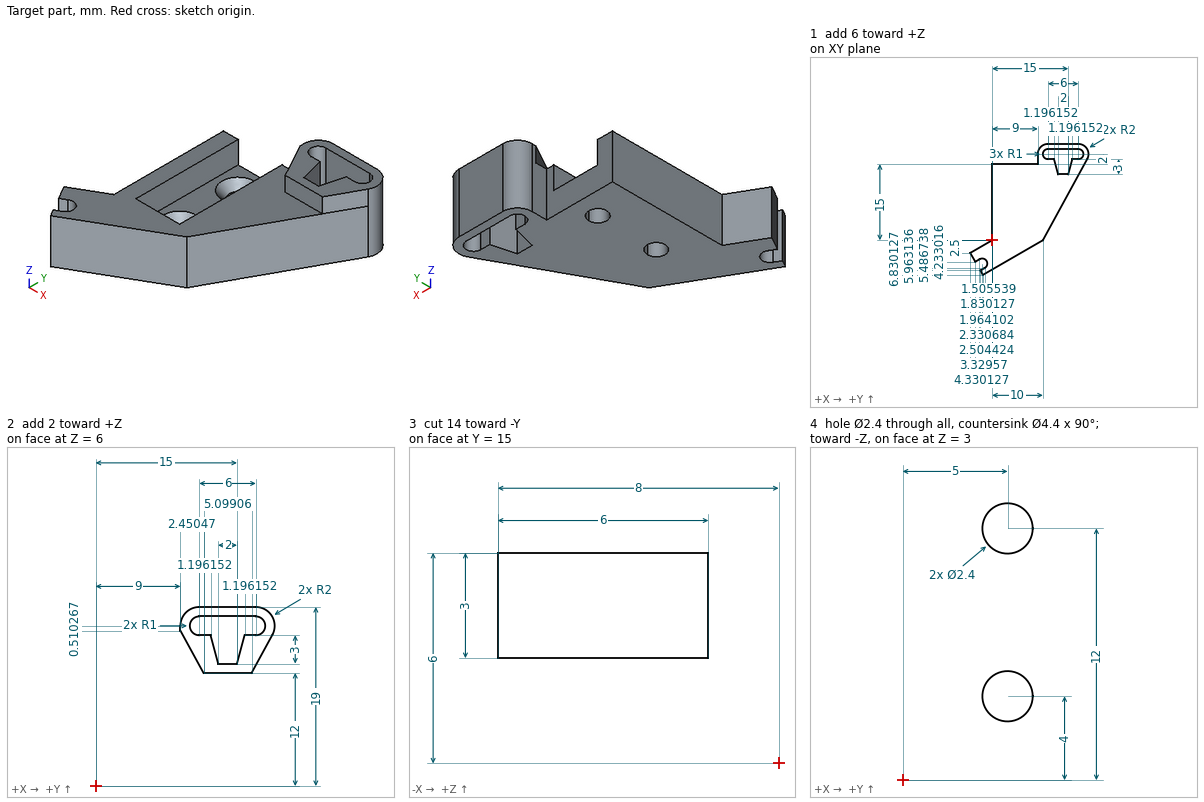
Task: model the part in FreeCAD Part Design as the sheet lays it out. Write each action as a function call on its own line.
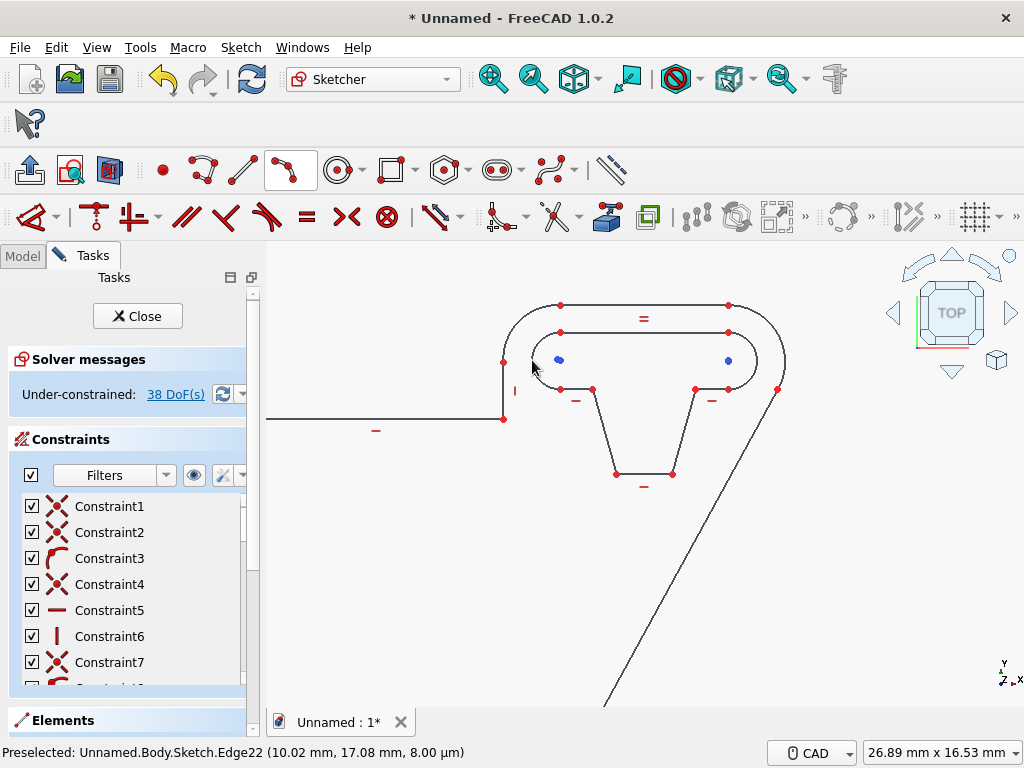
click(704, 524)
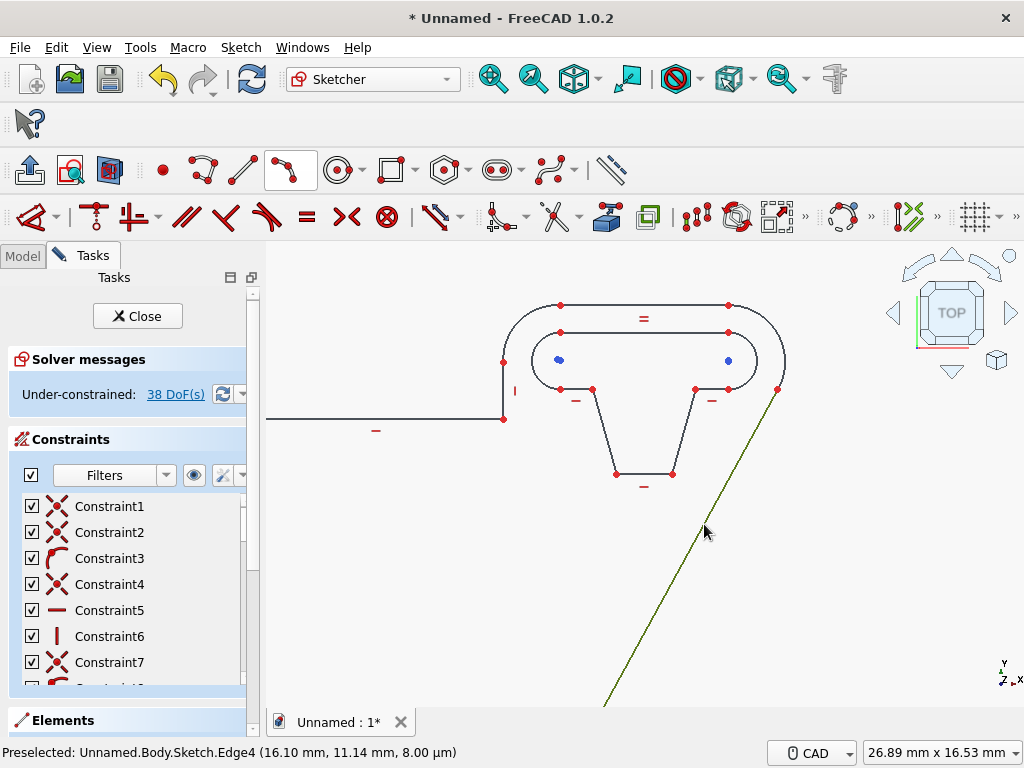
click(785, 356)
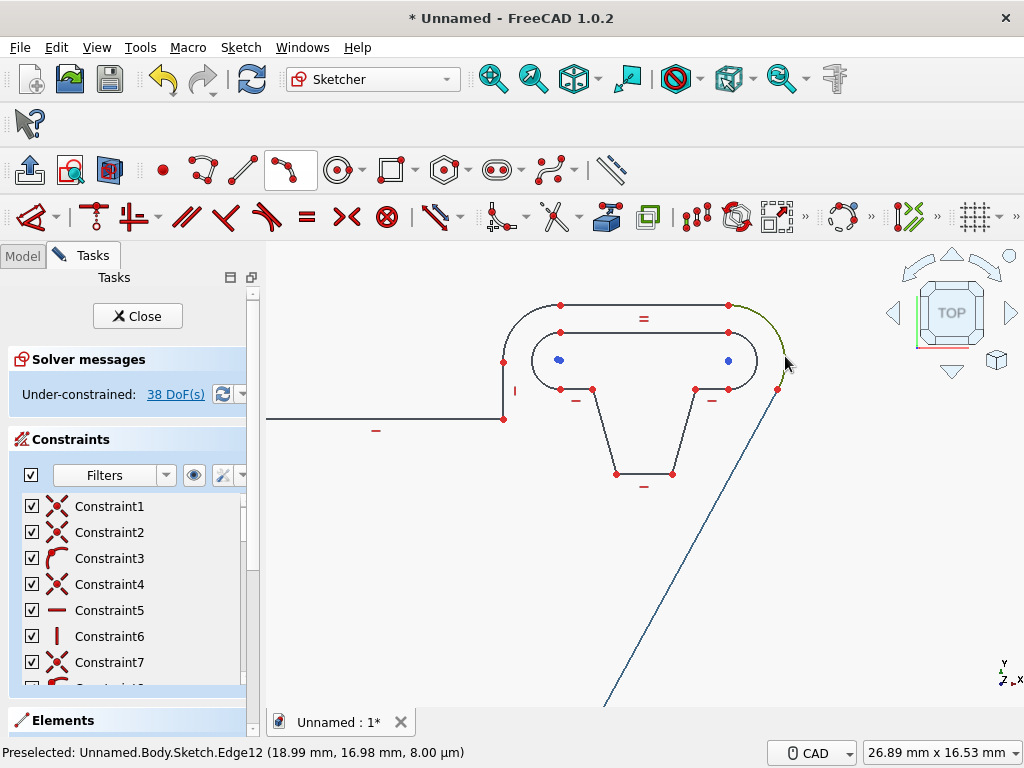
key(t)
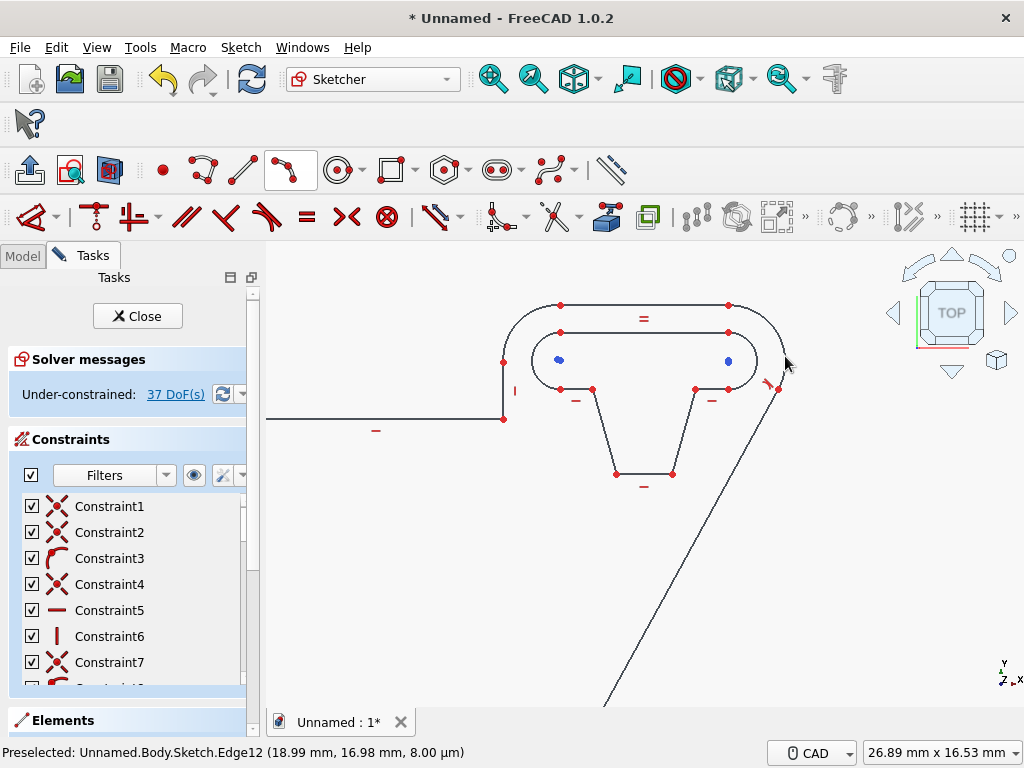
click(678, 305)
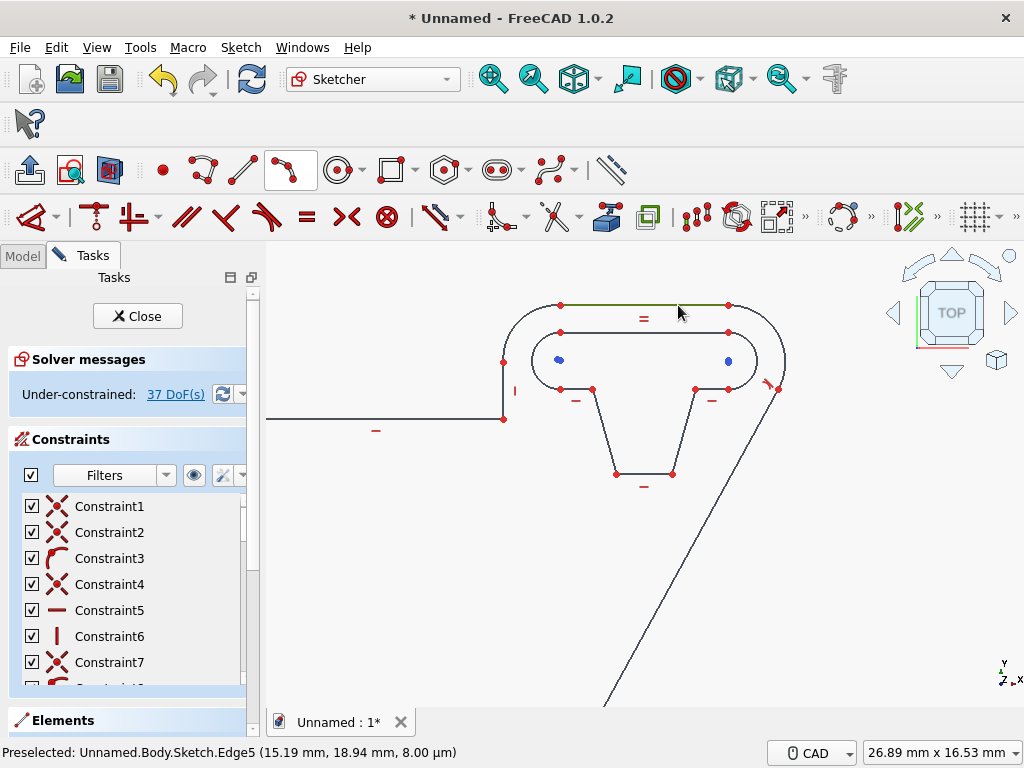
click(785, 355)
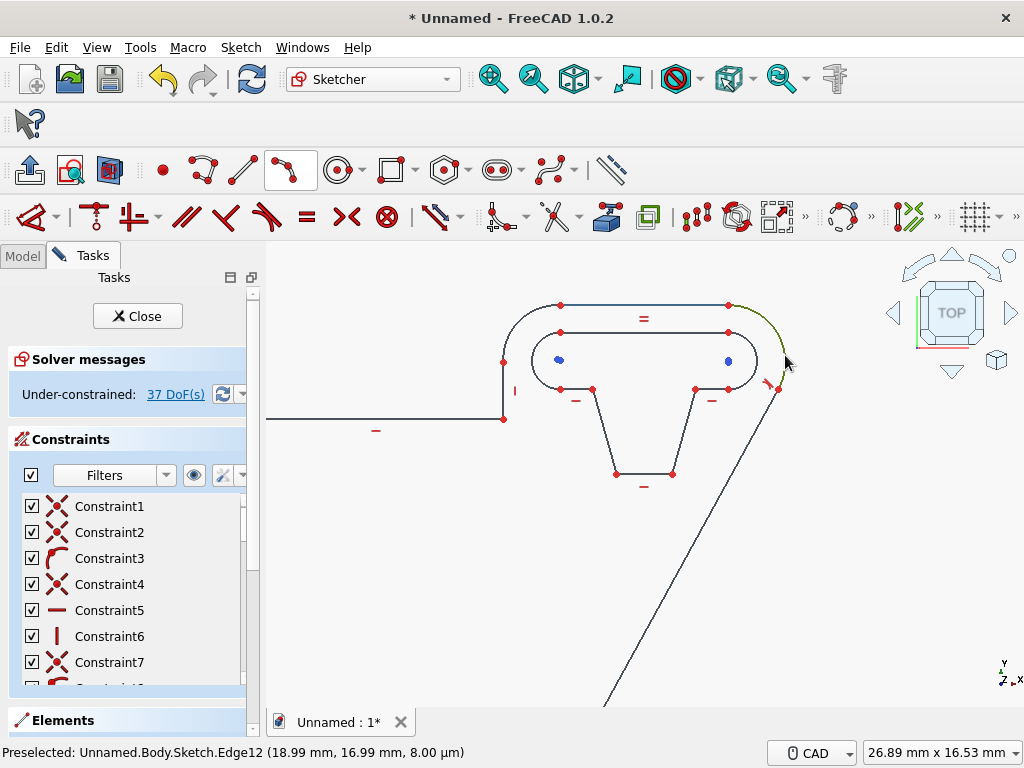
click(268, 218)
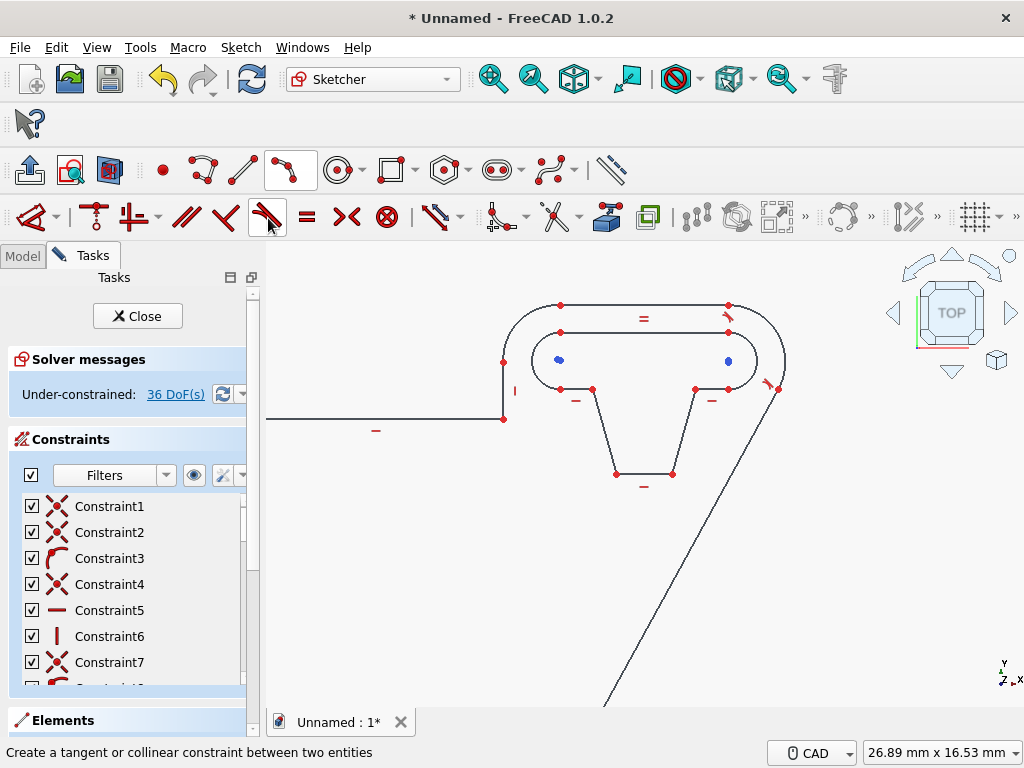
click(678, 305)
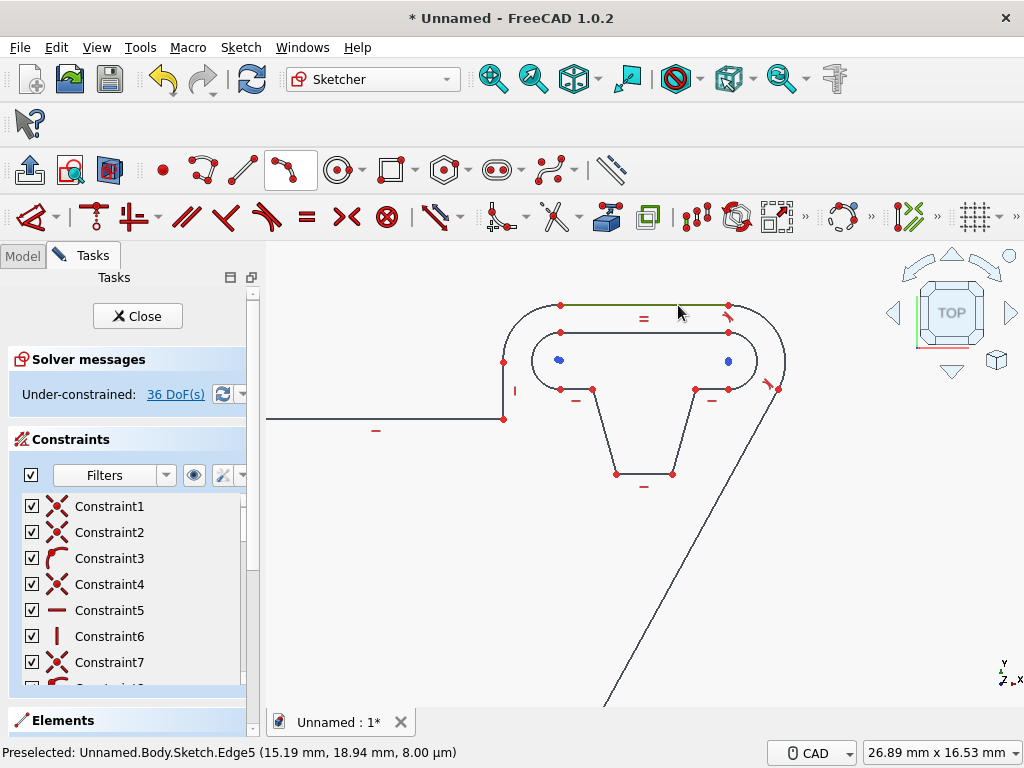
click(534, 311)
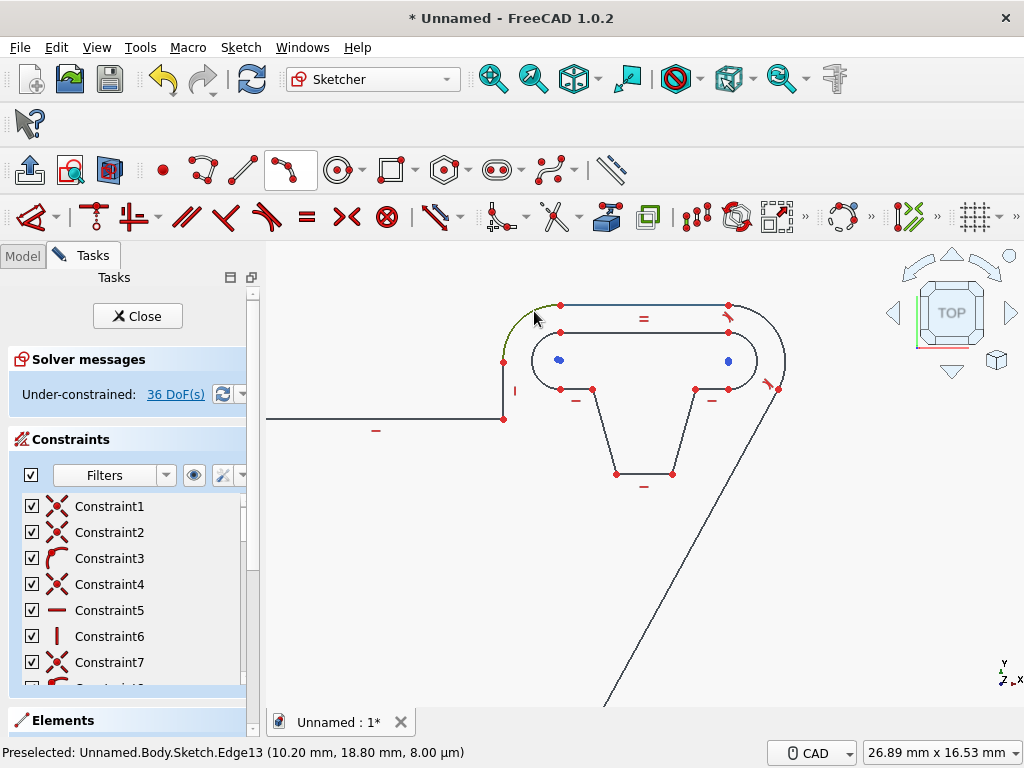
click(268, 218)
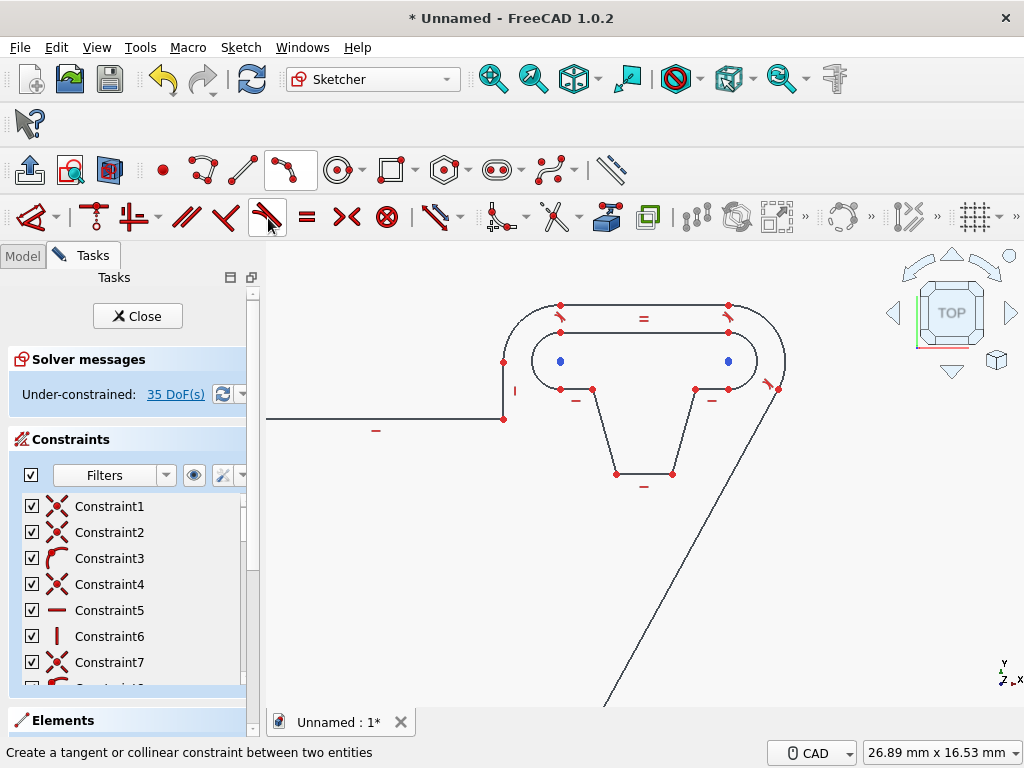
click(503, 379)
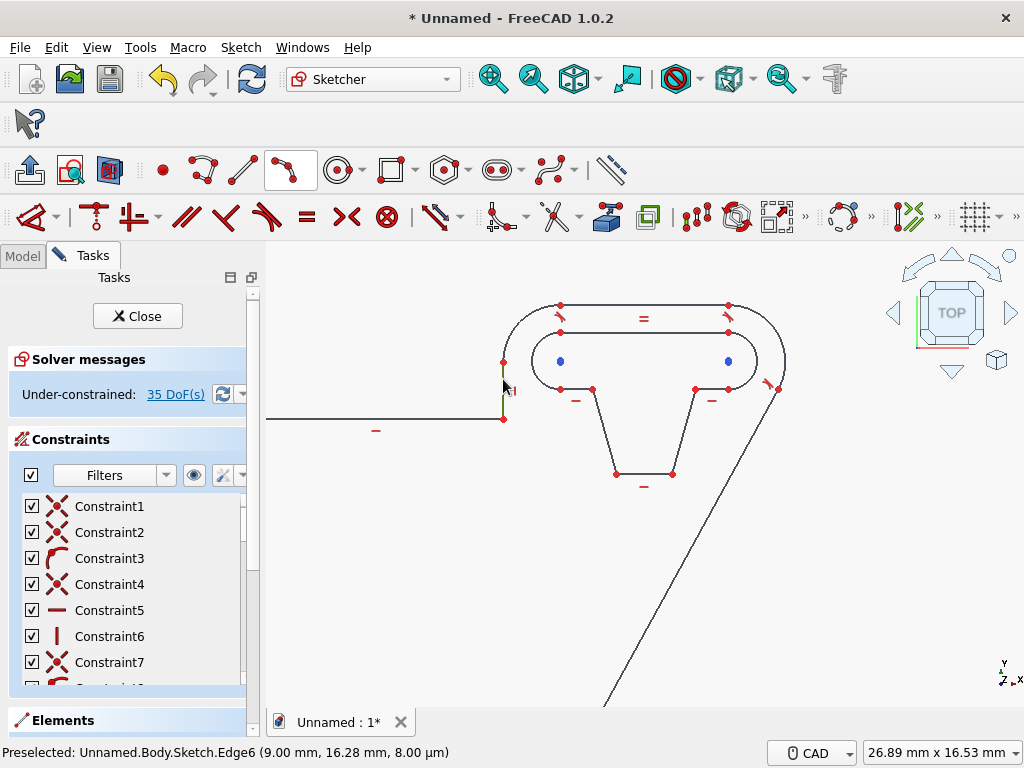
click(534, 311)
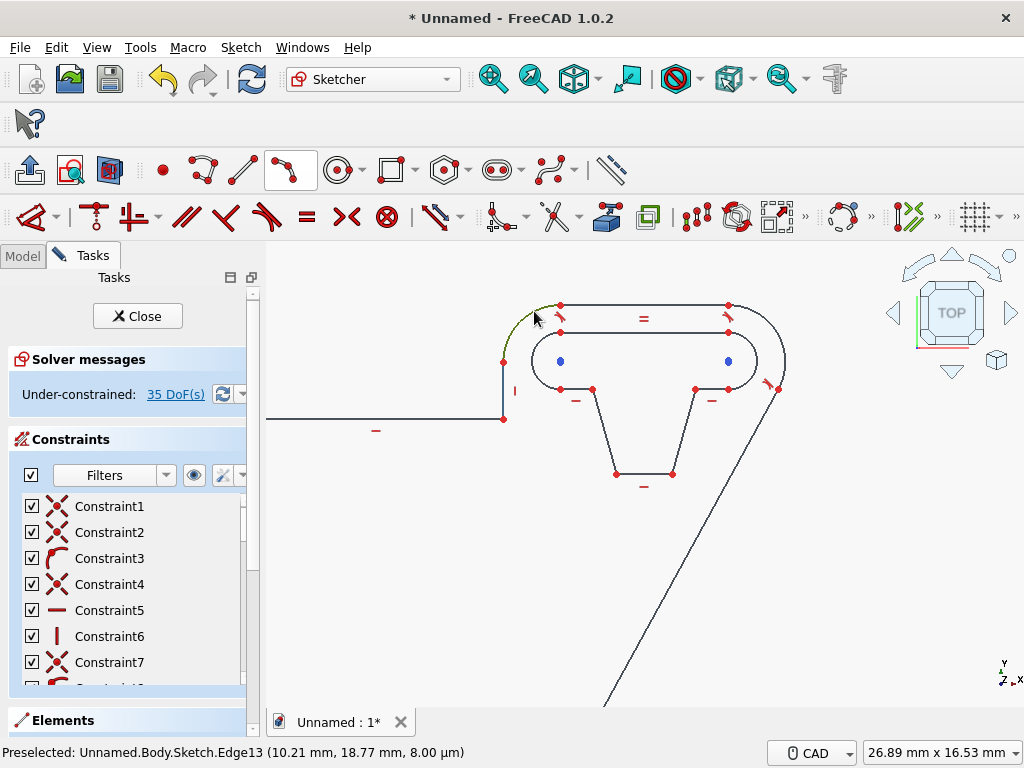
click(268, 218)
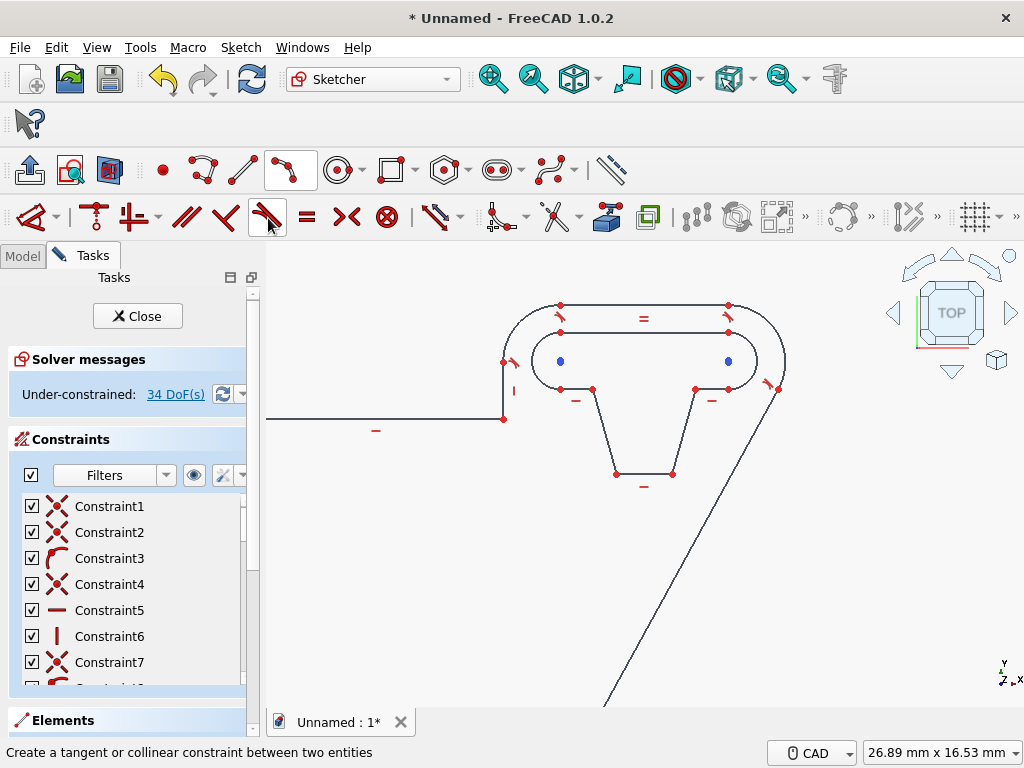
click(611, 333)